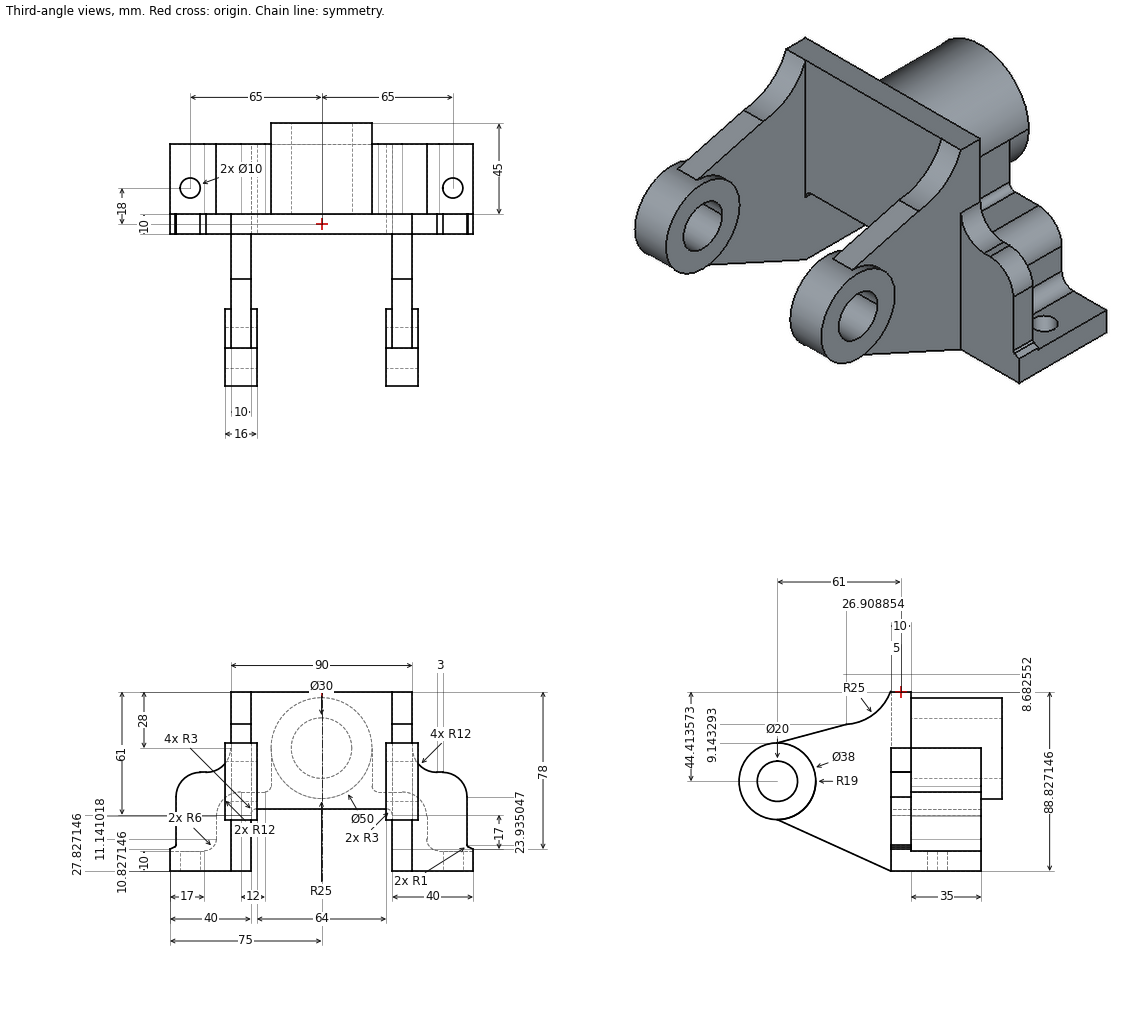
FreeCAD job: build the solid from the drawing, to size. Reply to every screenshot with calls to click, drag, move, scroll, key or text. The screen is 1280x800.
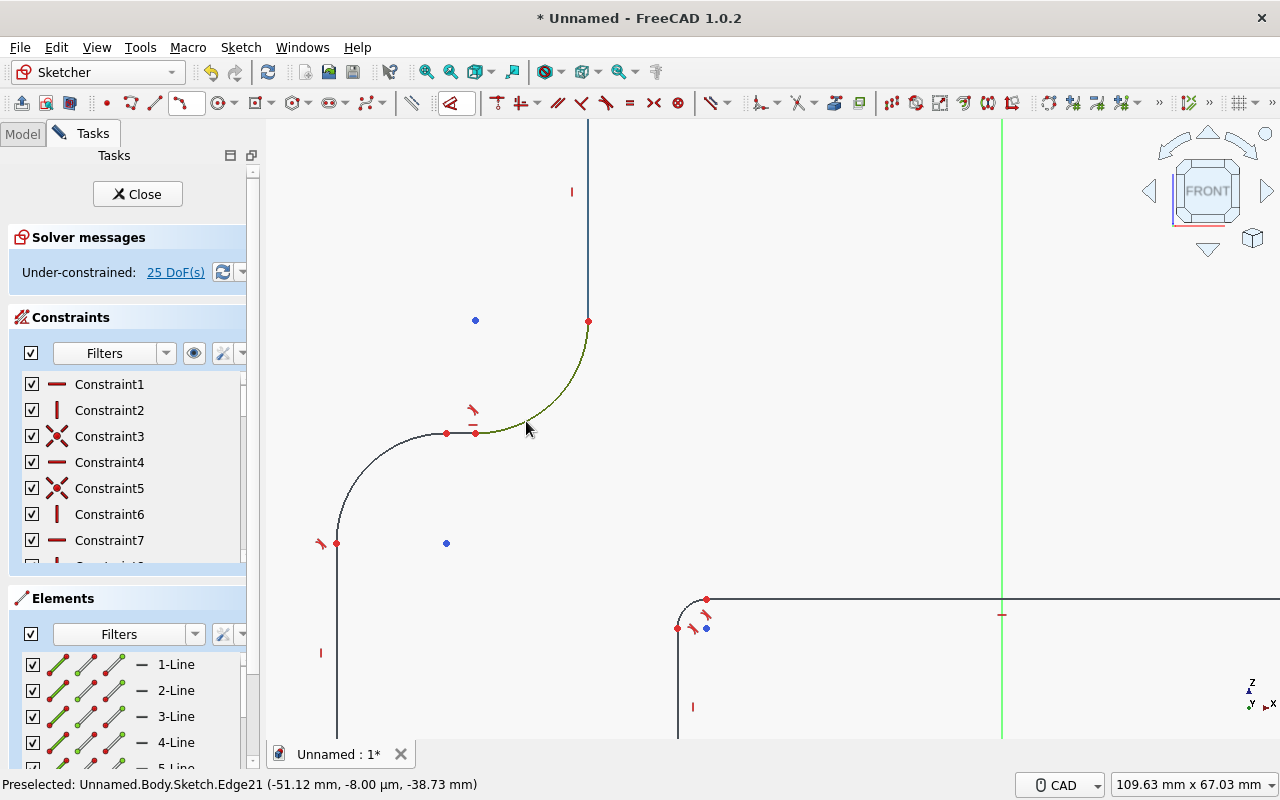
click(606, 104)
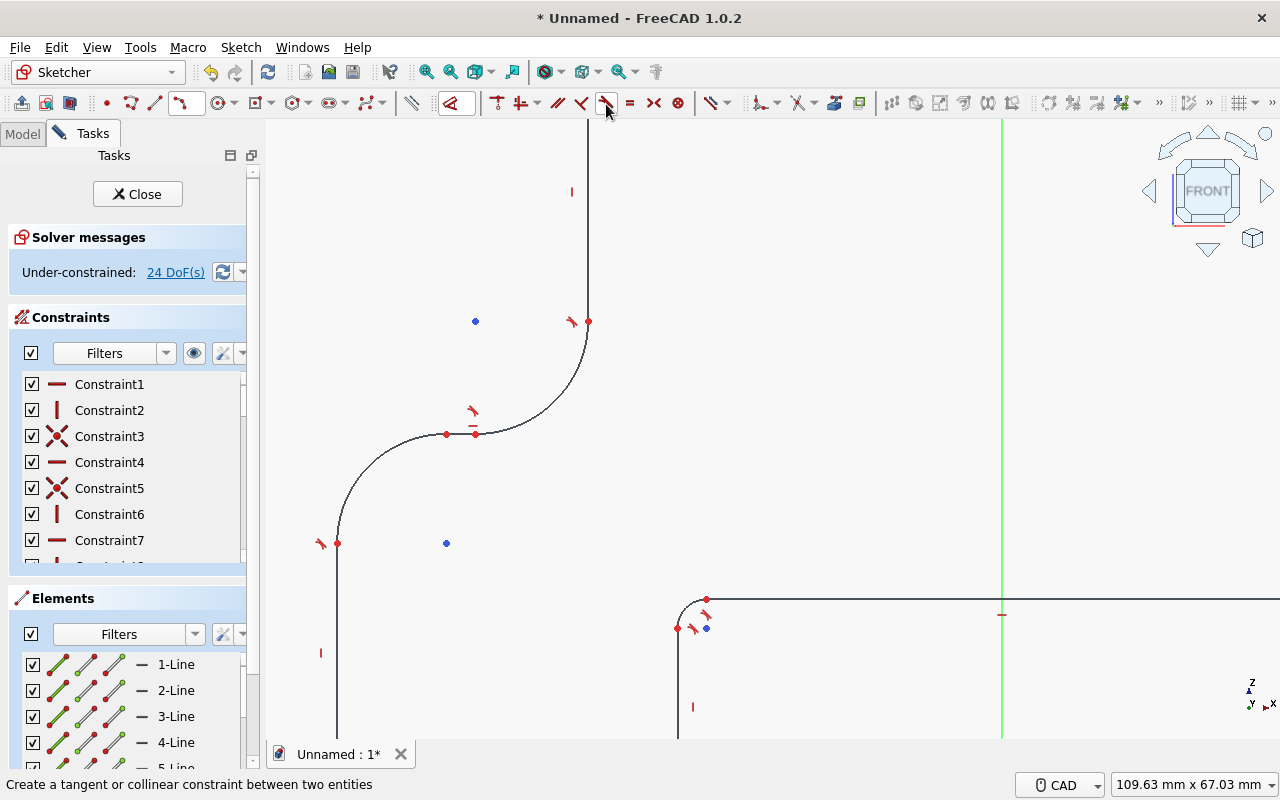
scroll(462, 435, down, 4)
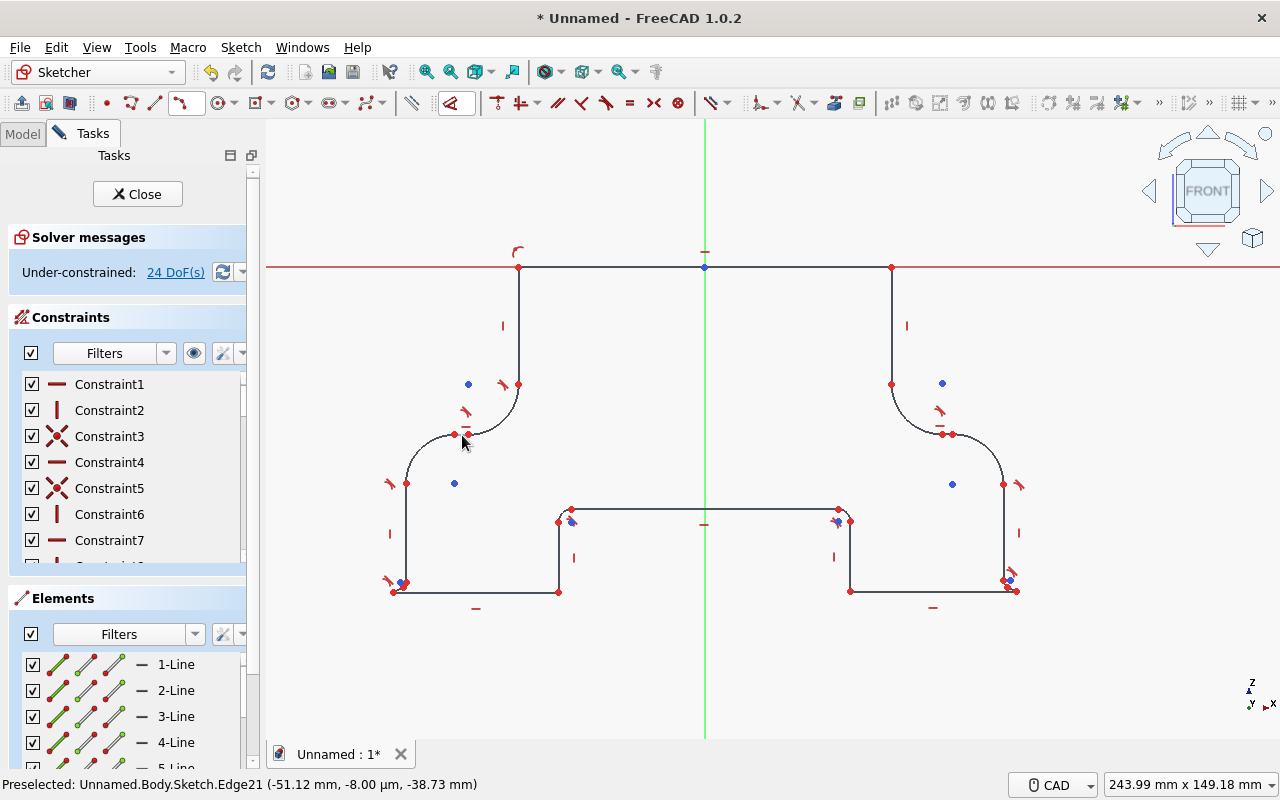
click(892, 302)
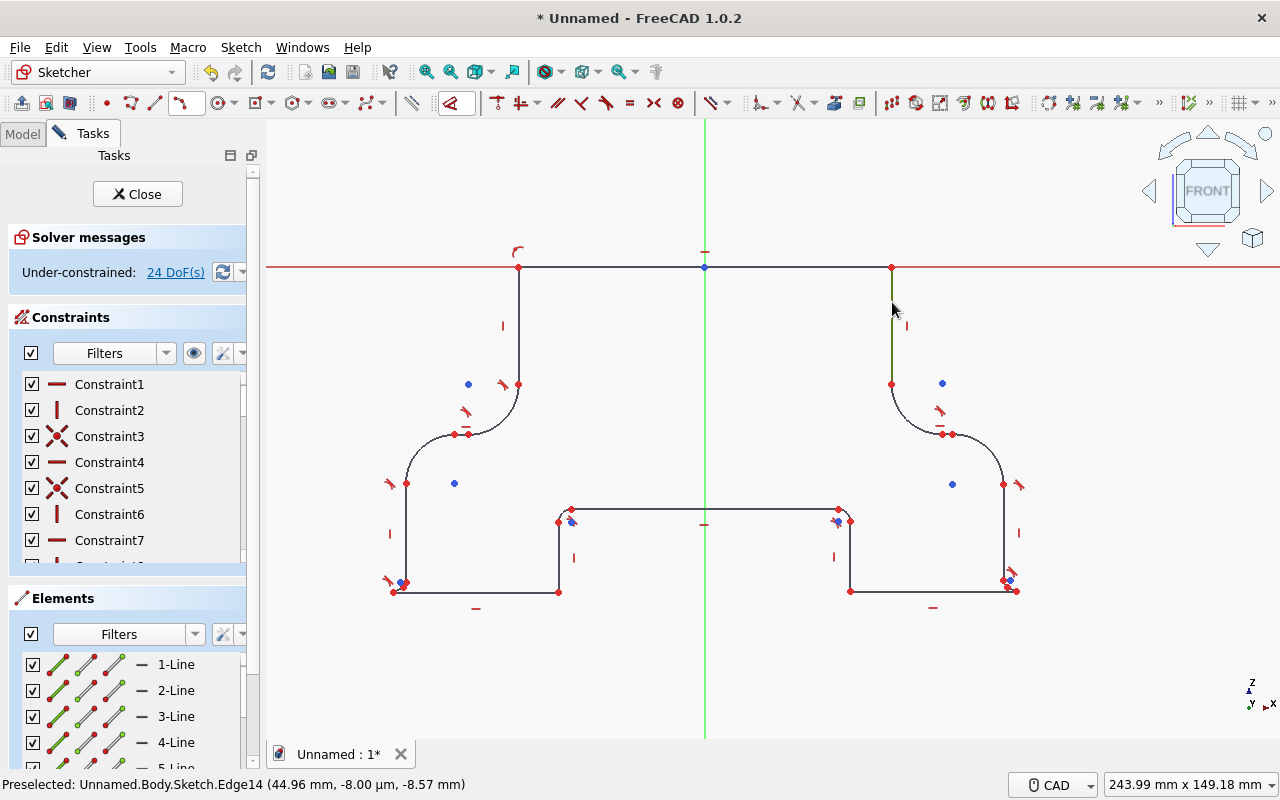
click(897, 407)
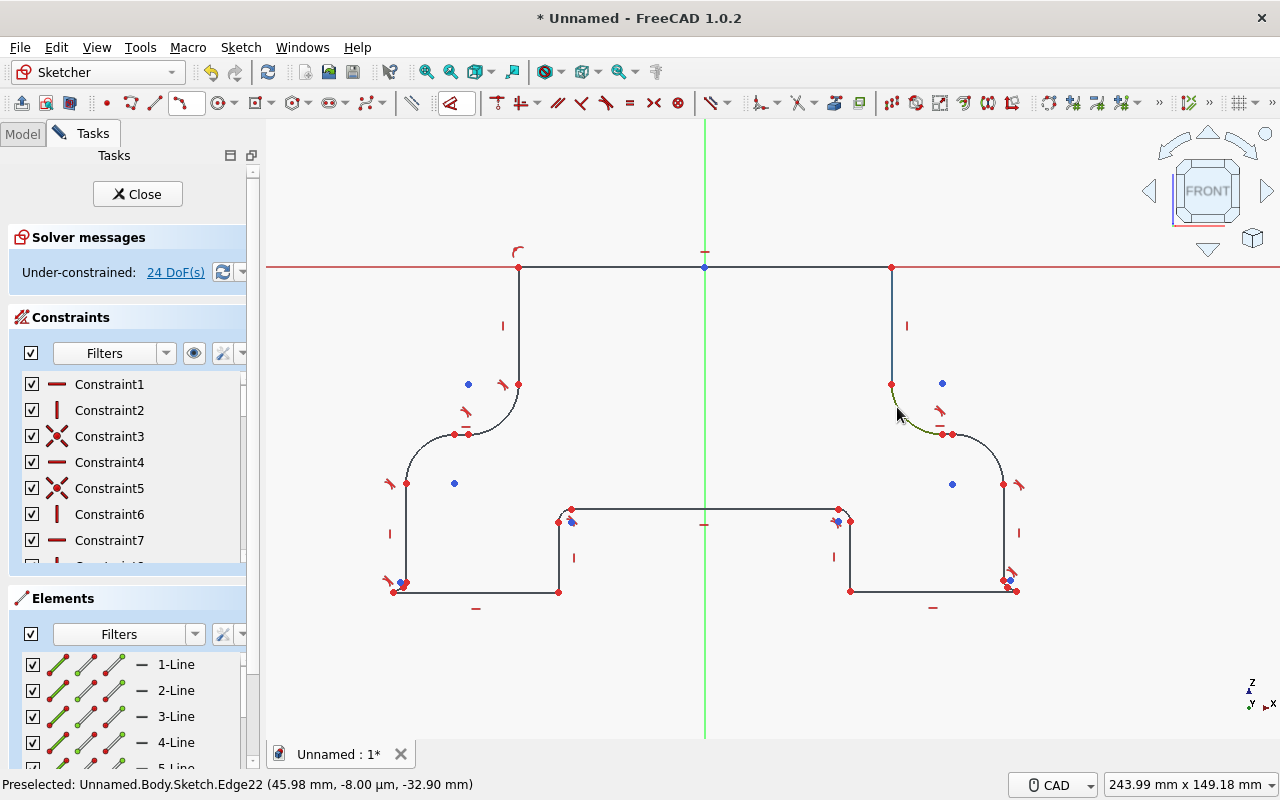
click(606, 104)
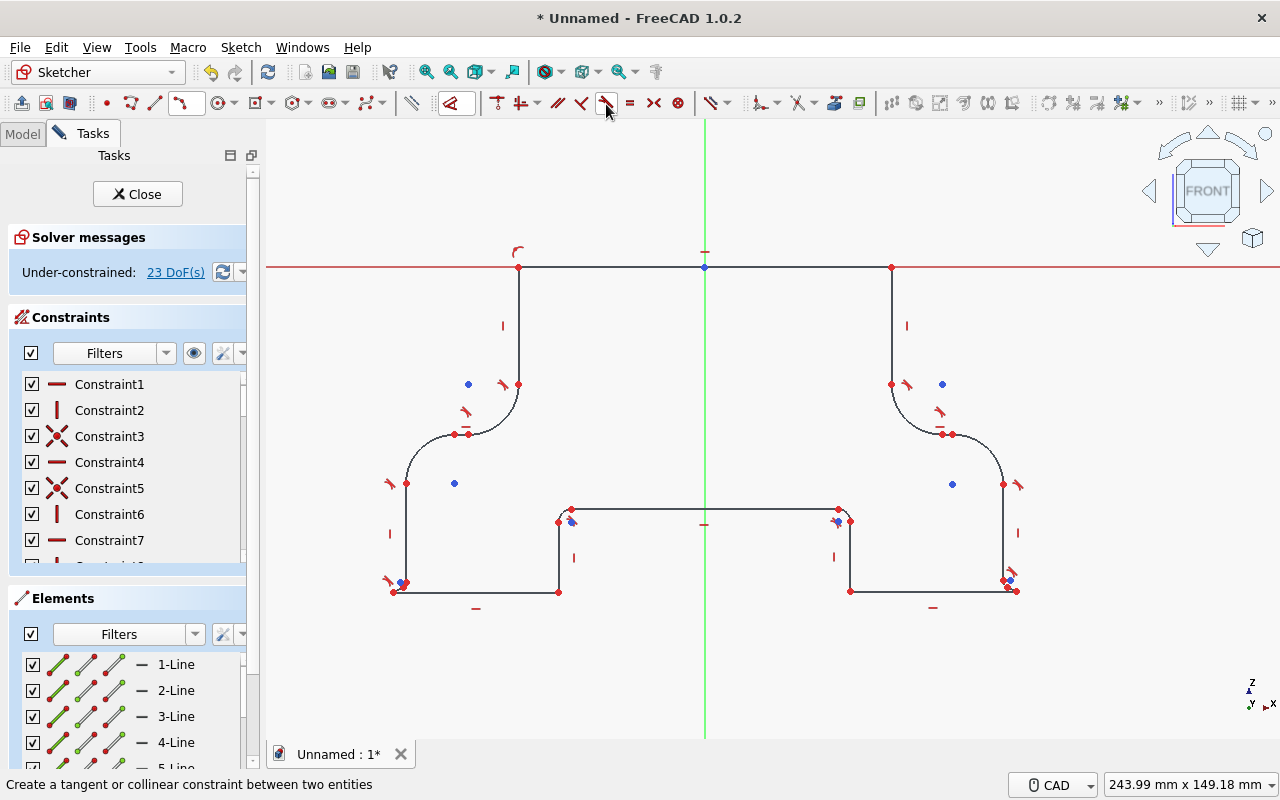
scroll(847, 513, up, 2)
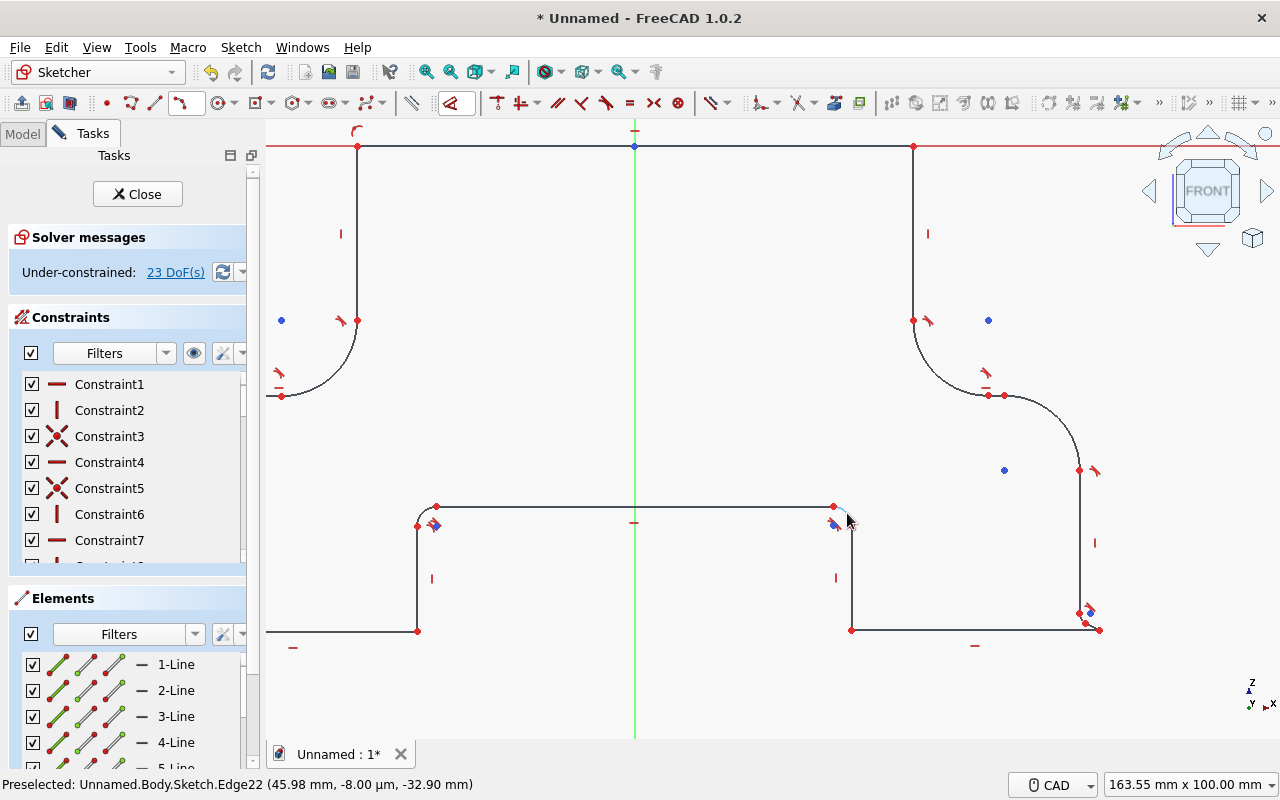
click(846, 512)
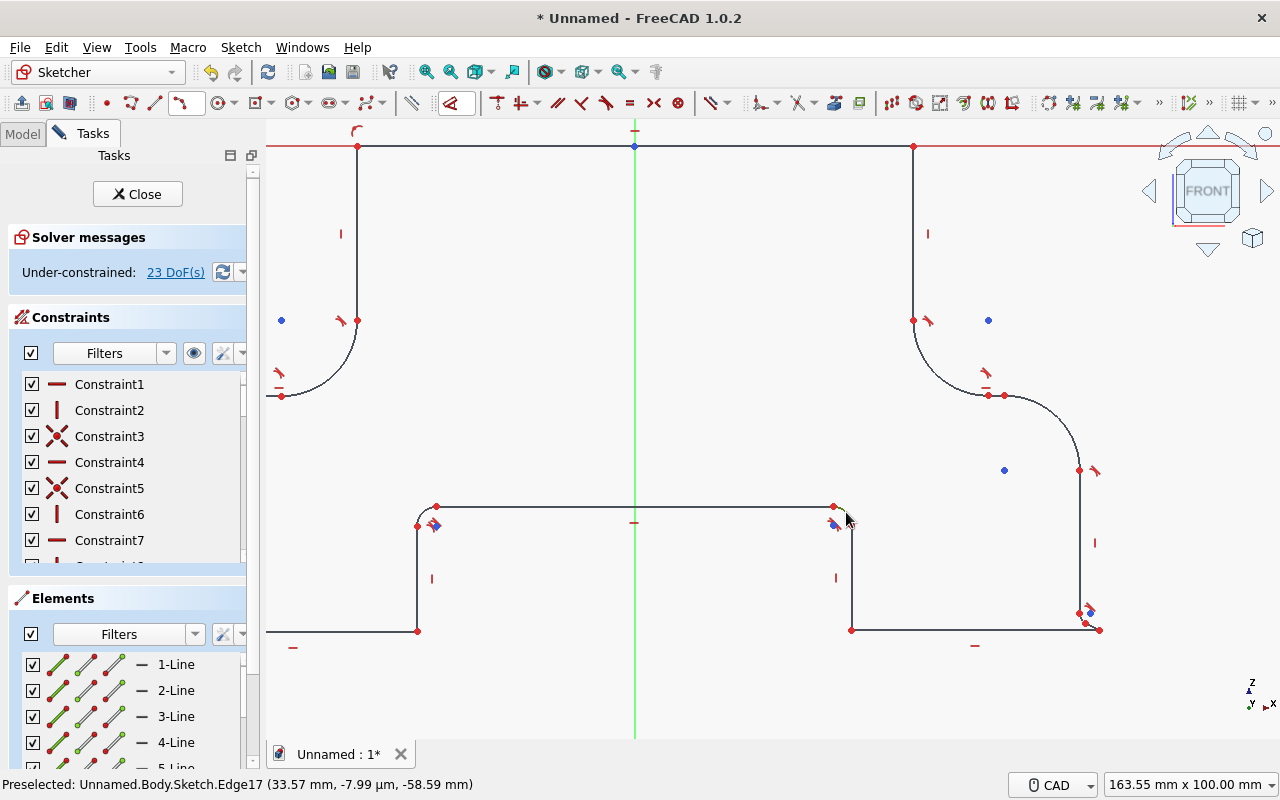
scroll(428, 509, up, 3)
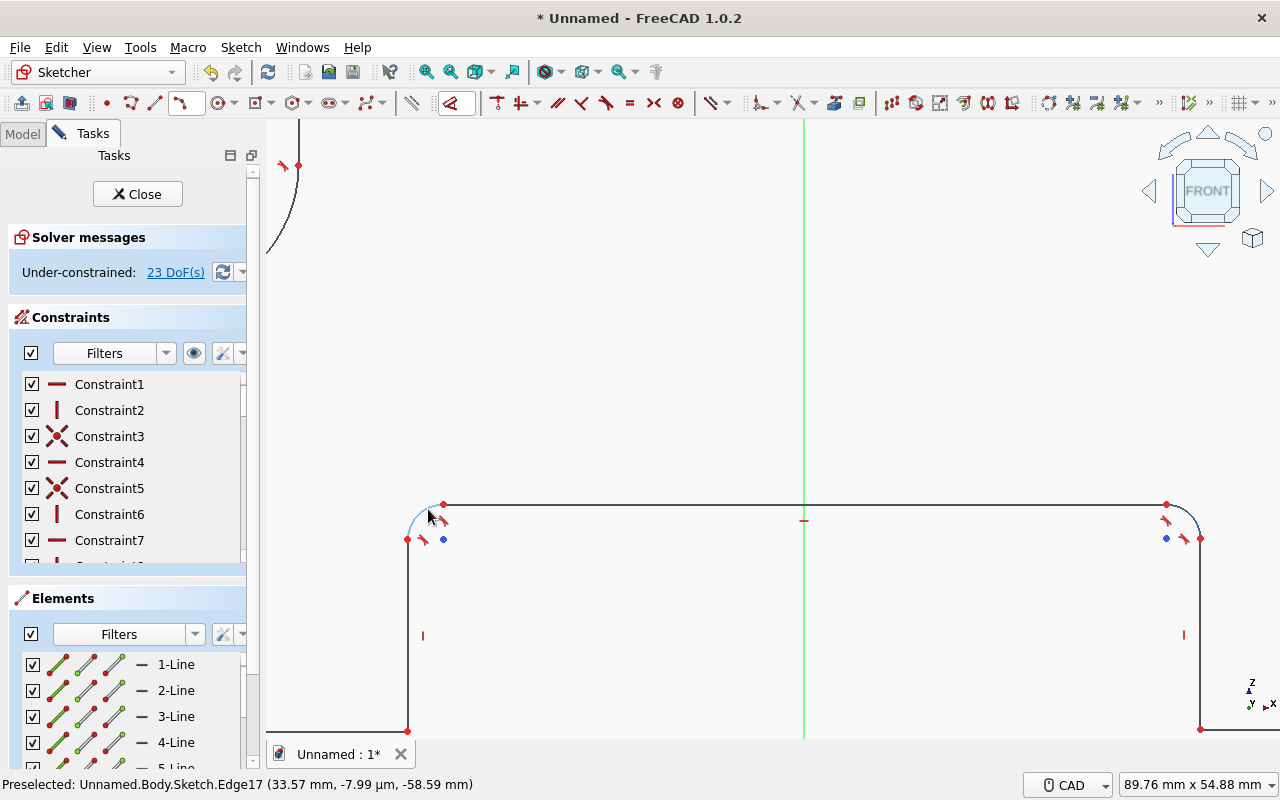
click(427, 509)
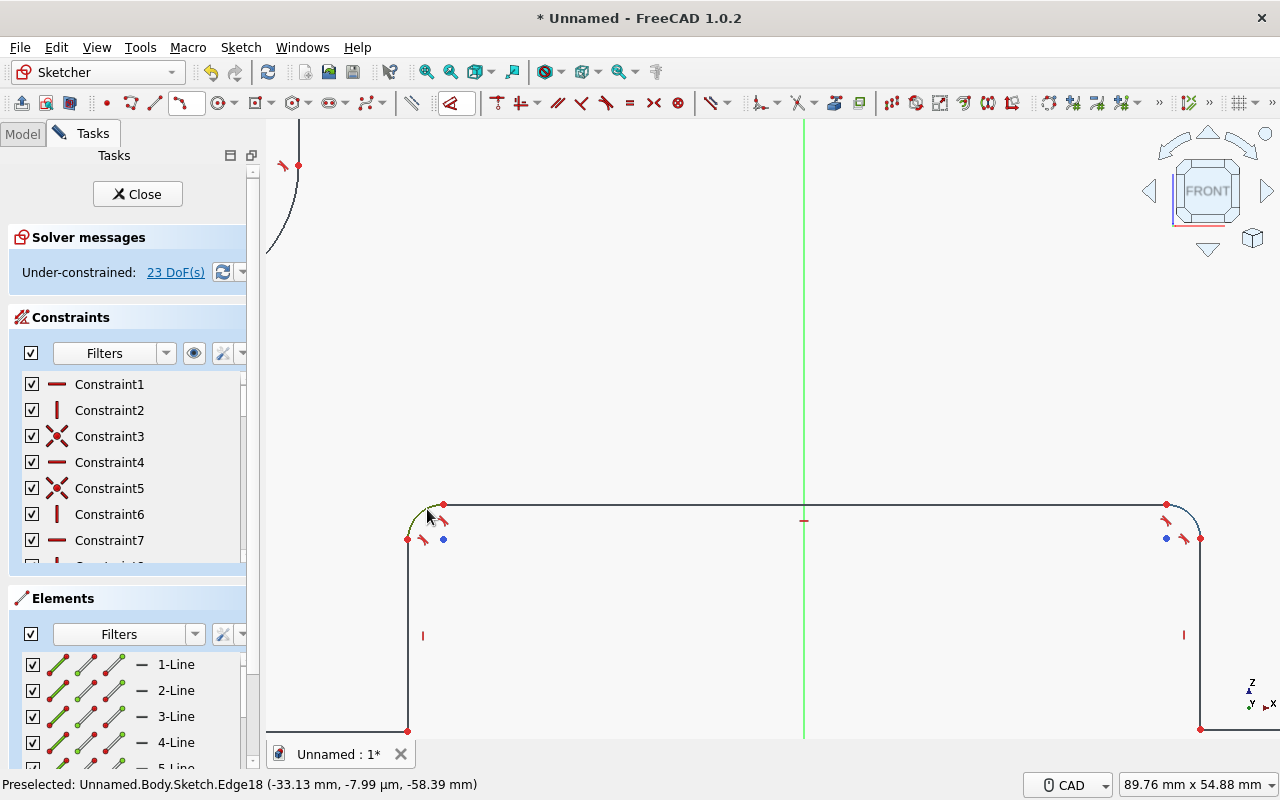
click(630, 104)